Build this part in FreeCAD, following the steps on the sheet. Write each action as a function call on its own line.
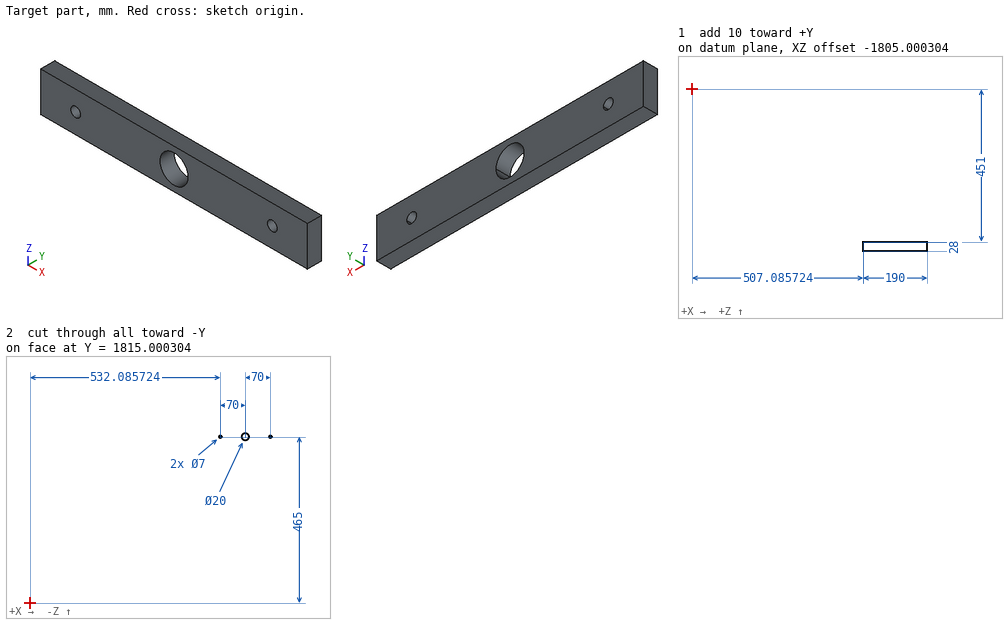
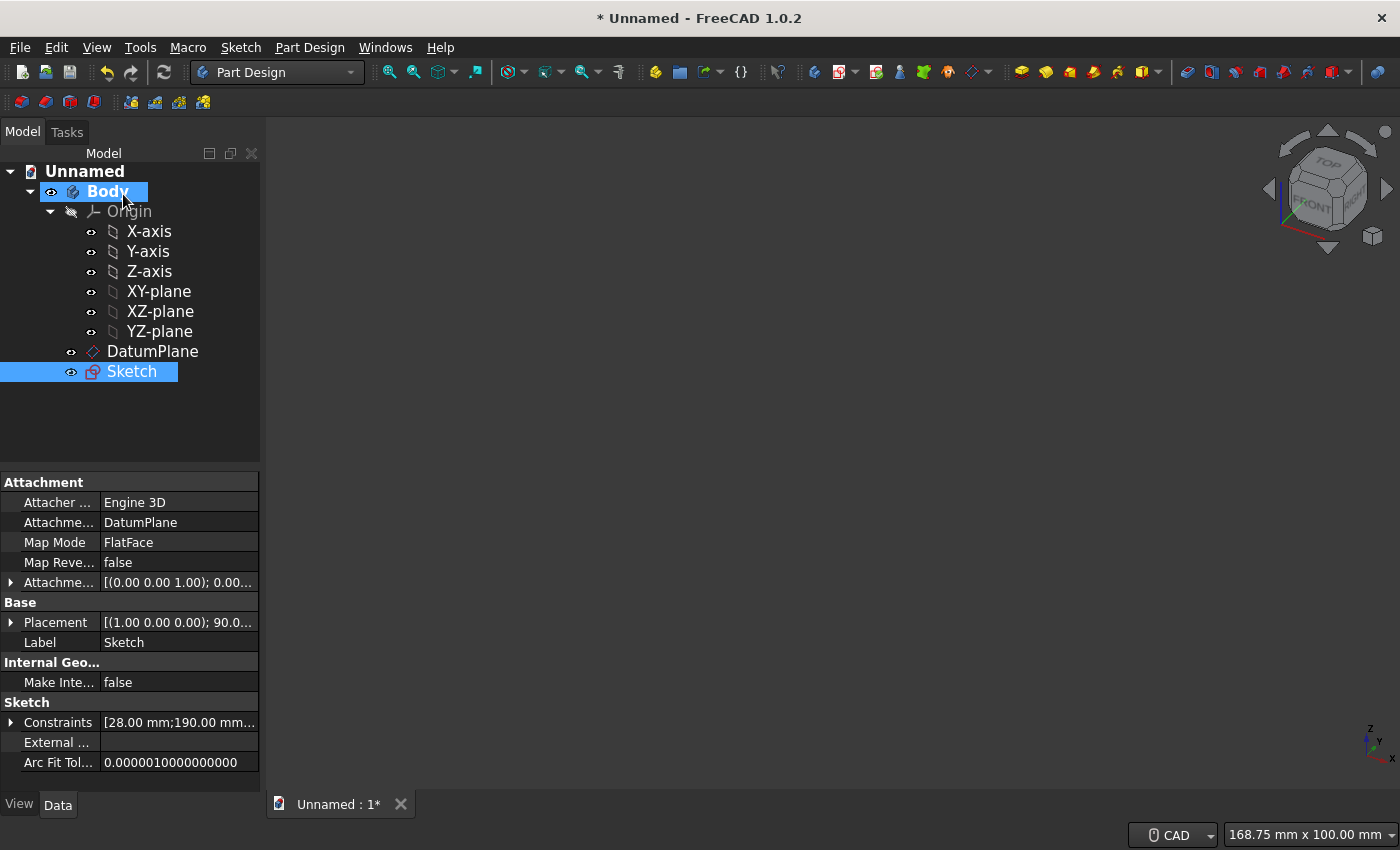
click(1022, 72)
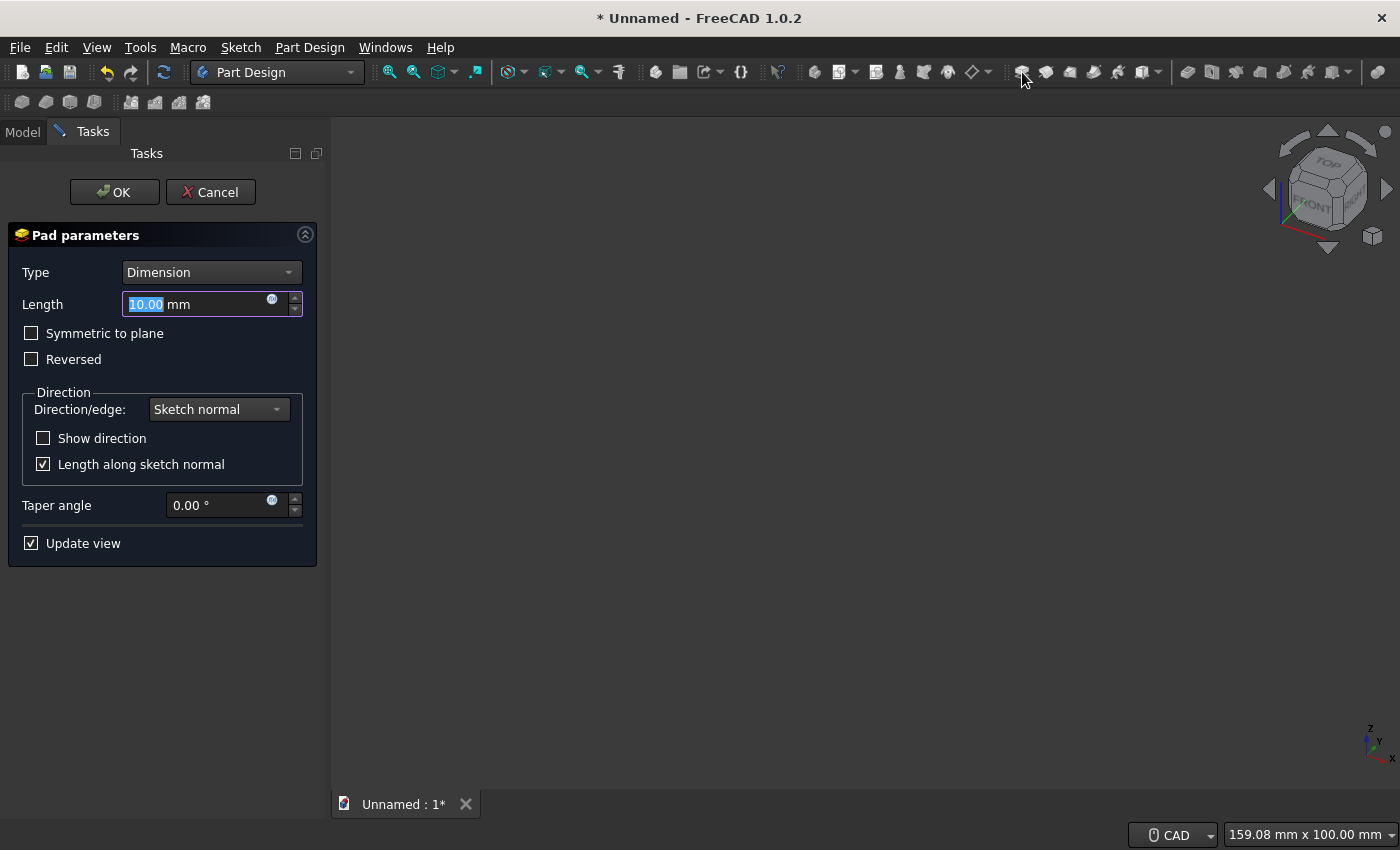
text(10)
key(Tab)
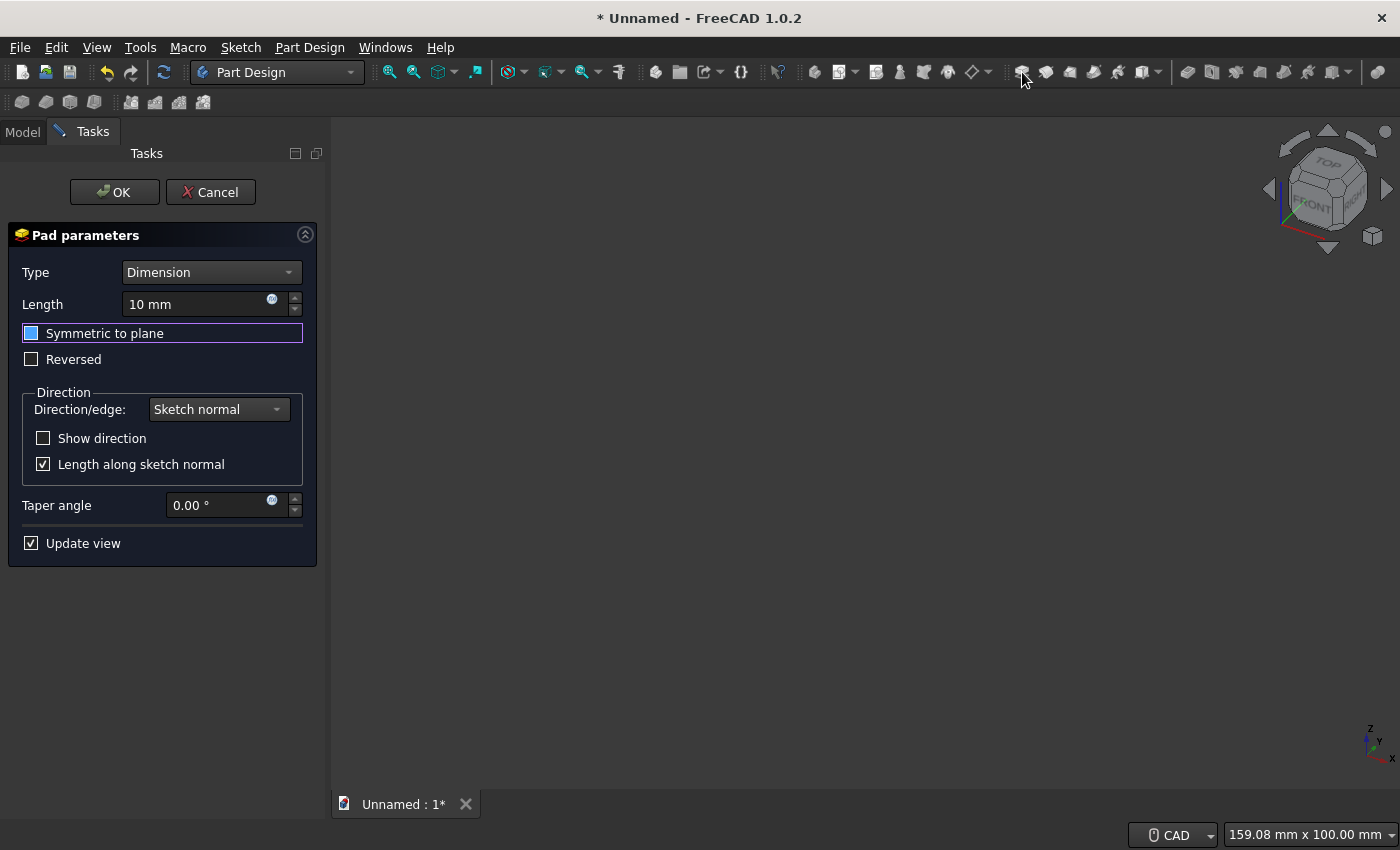
click(30, 359)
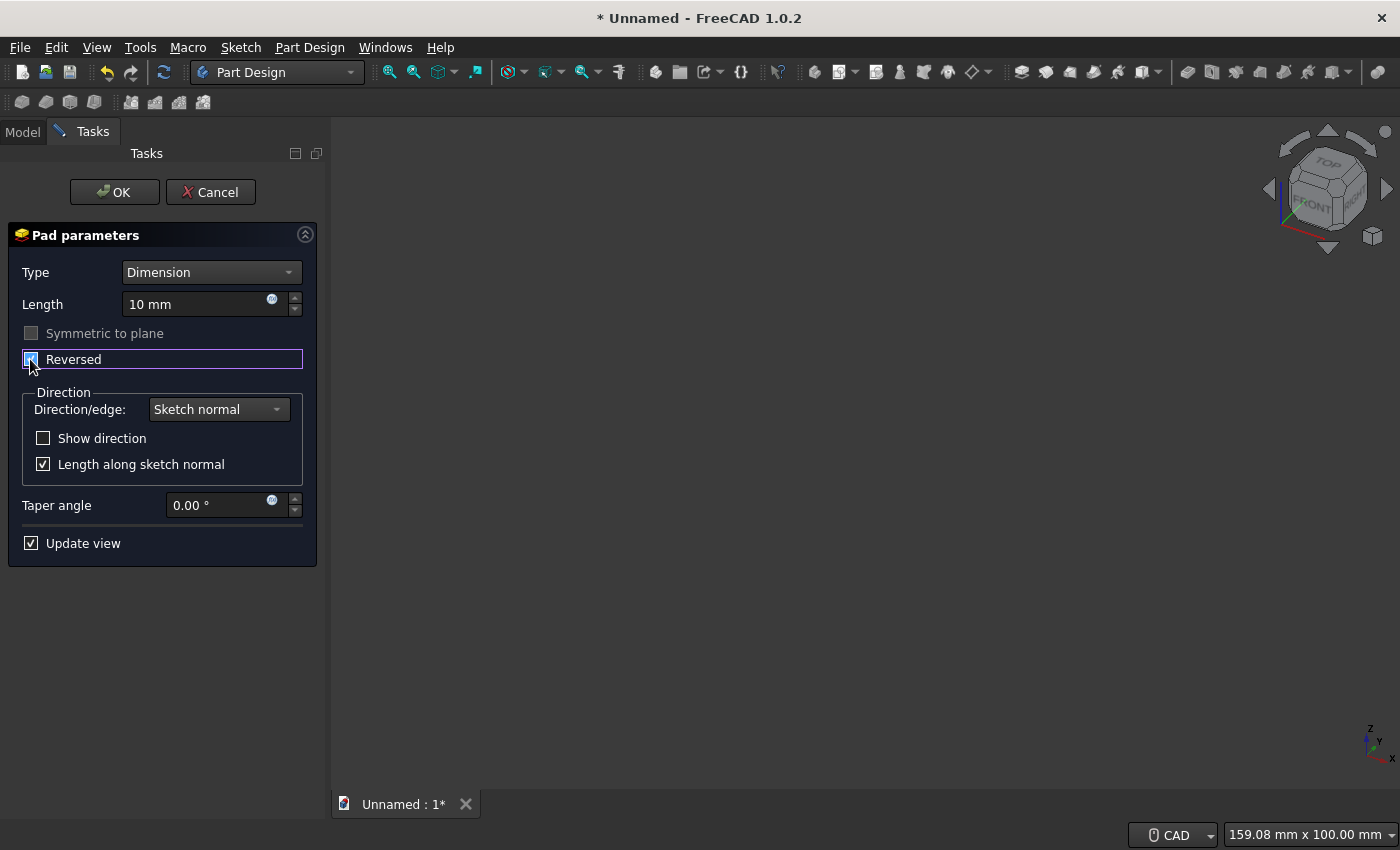
click(115, 192)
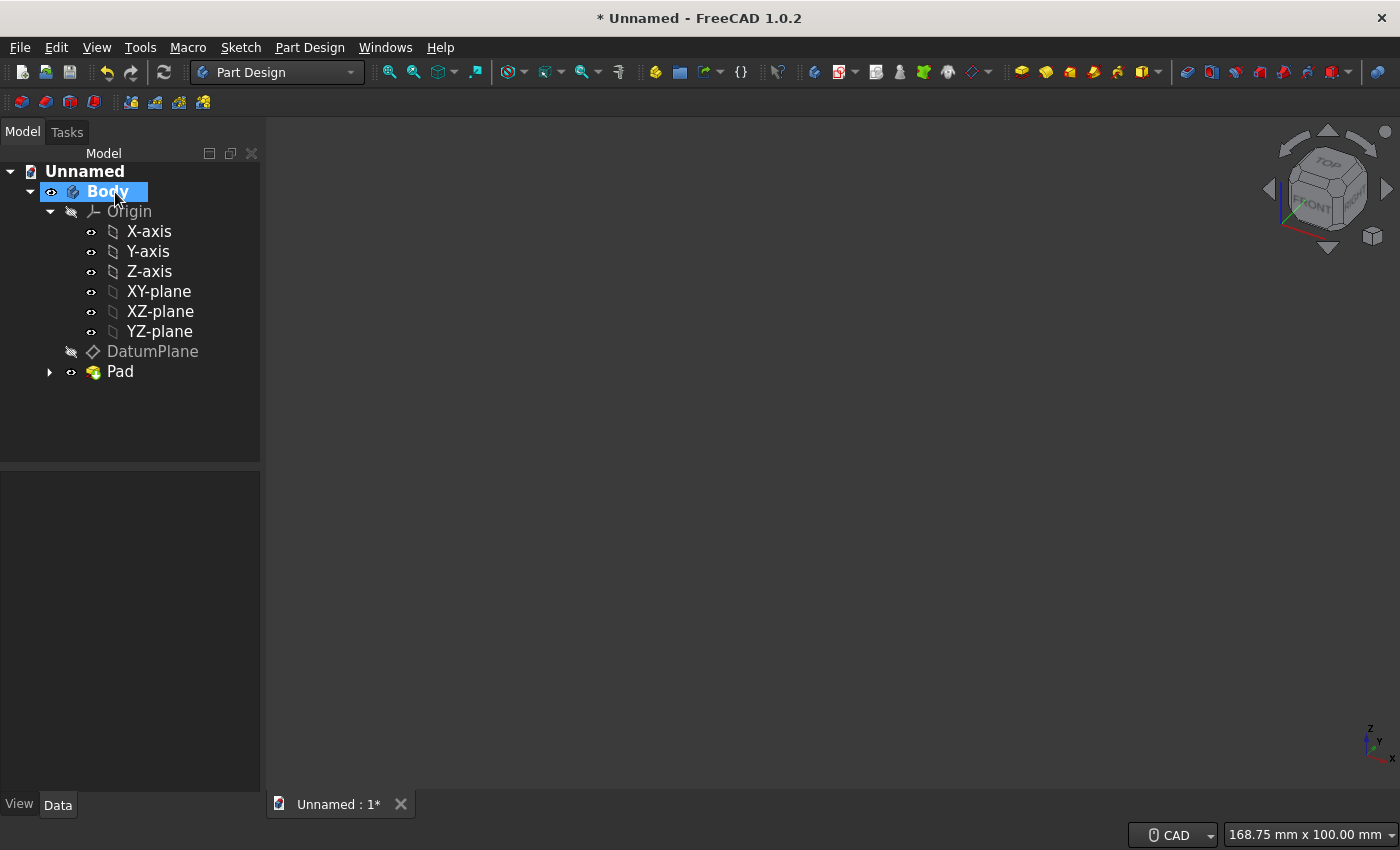
click(390, 72)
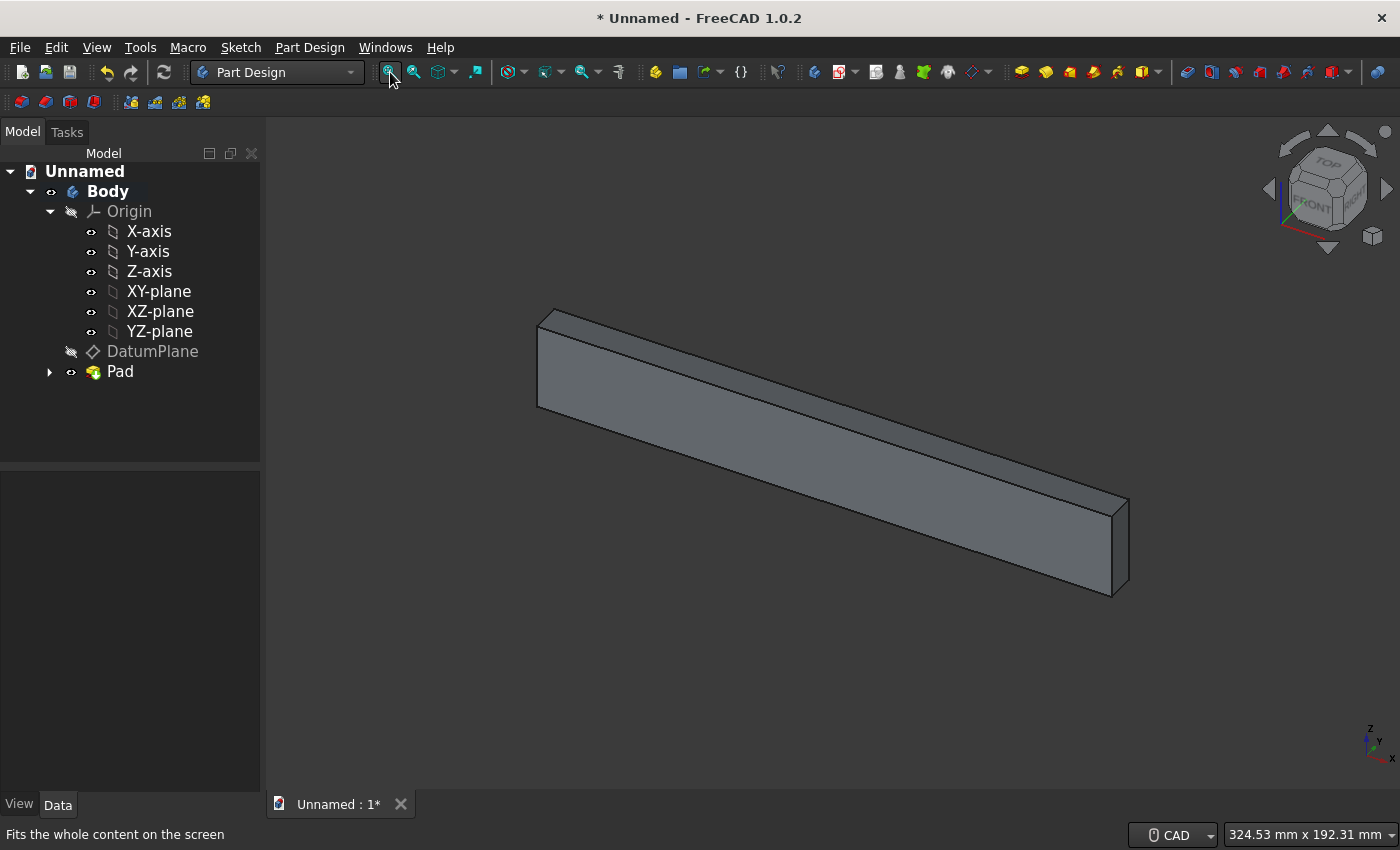
key(4)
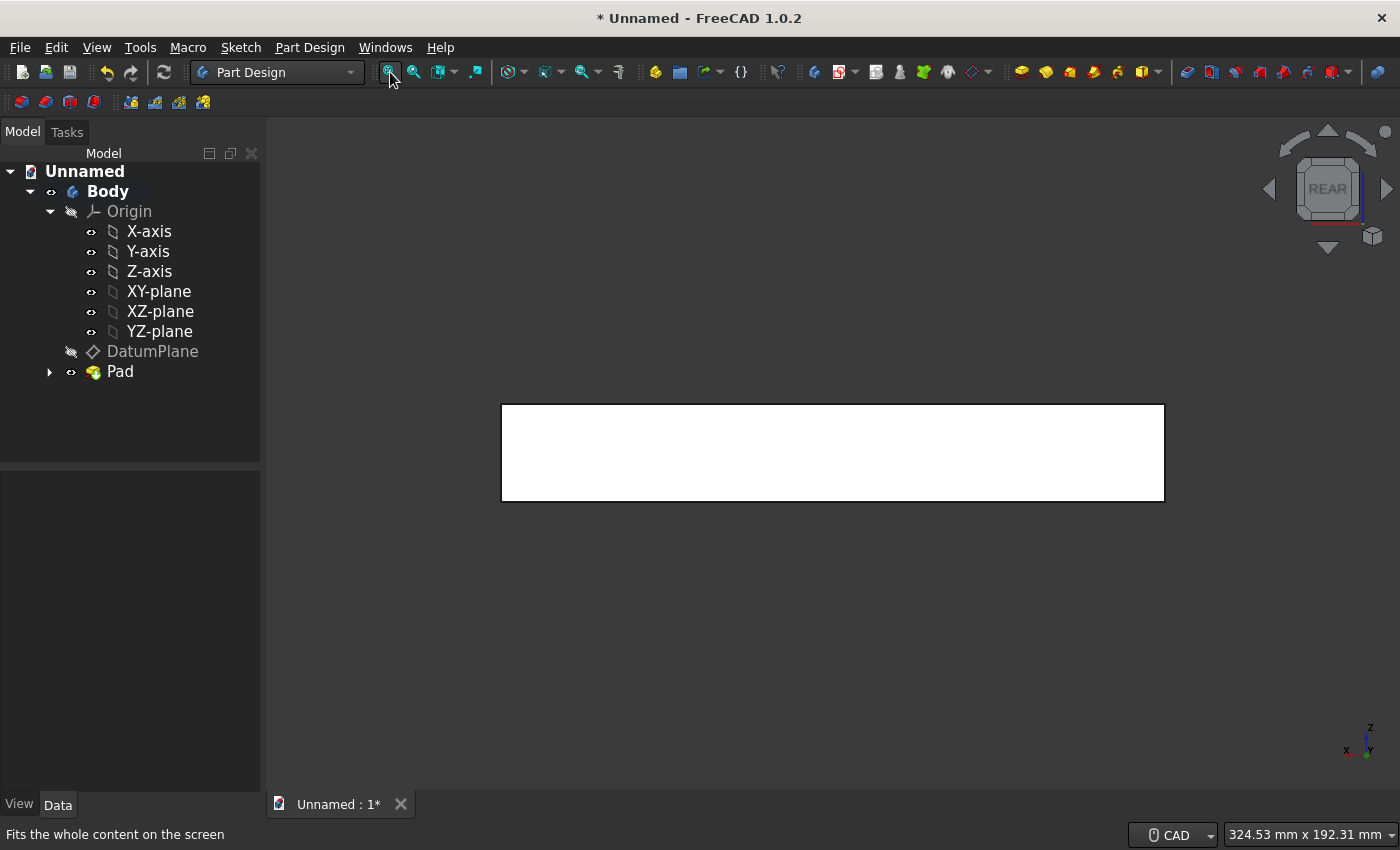
click(643, 452)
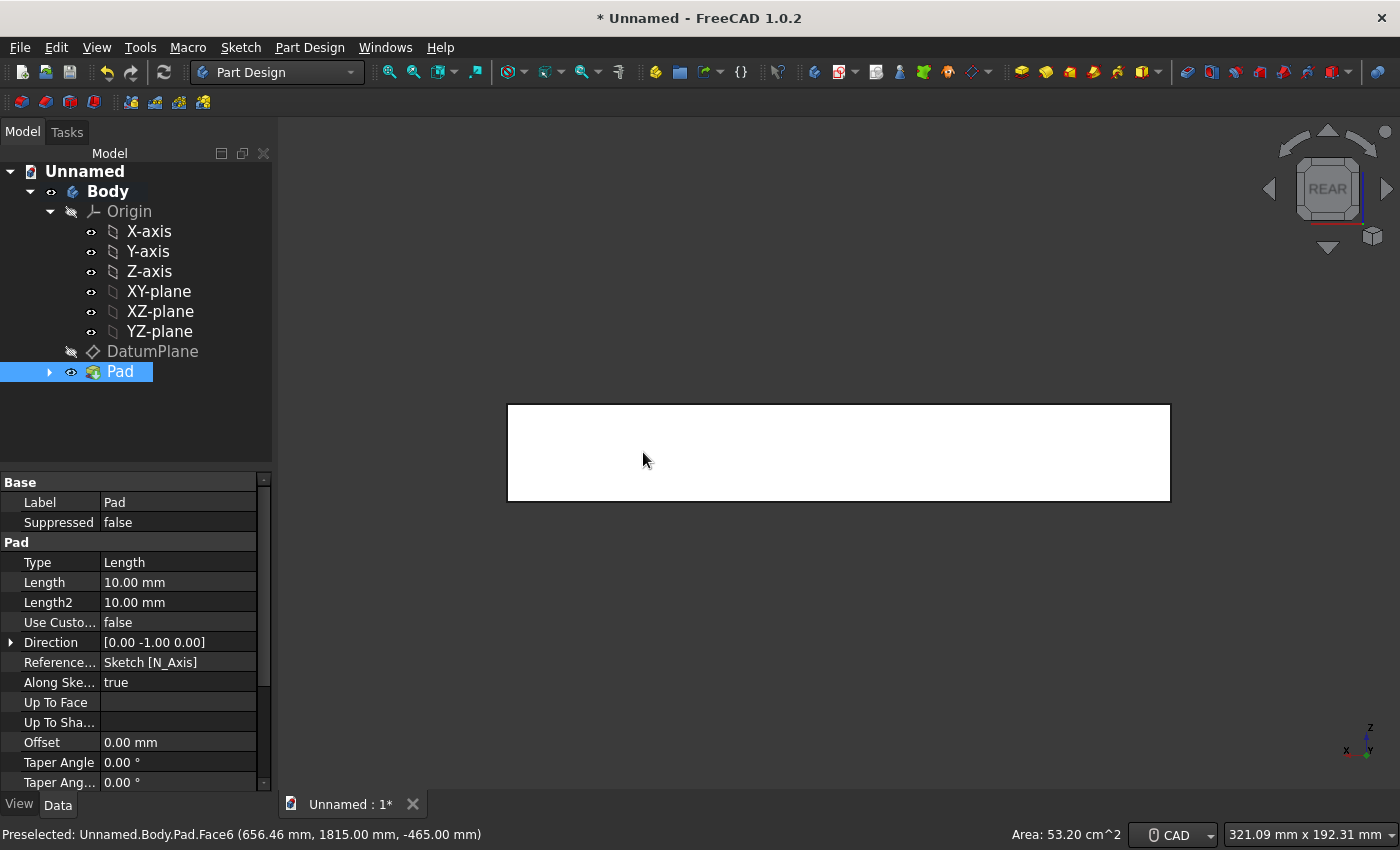
click(840, 72)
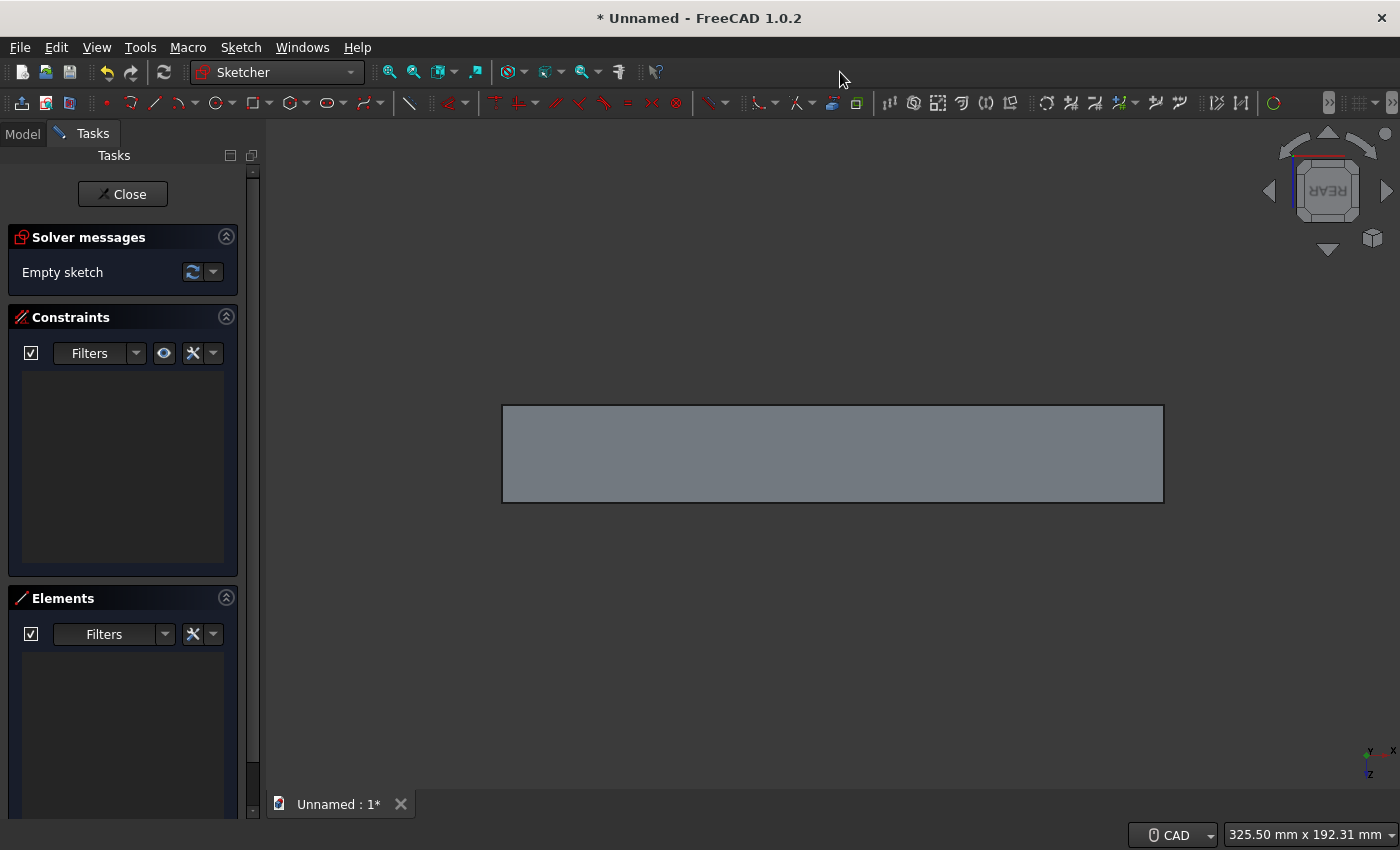
click(216, 104)